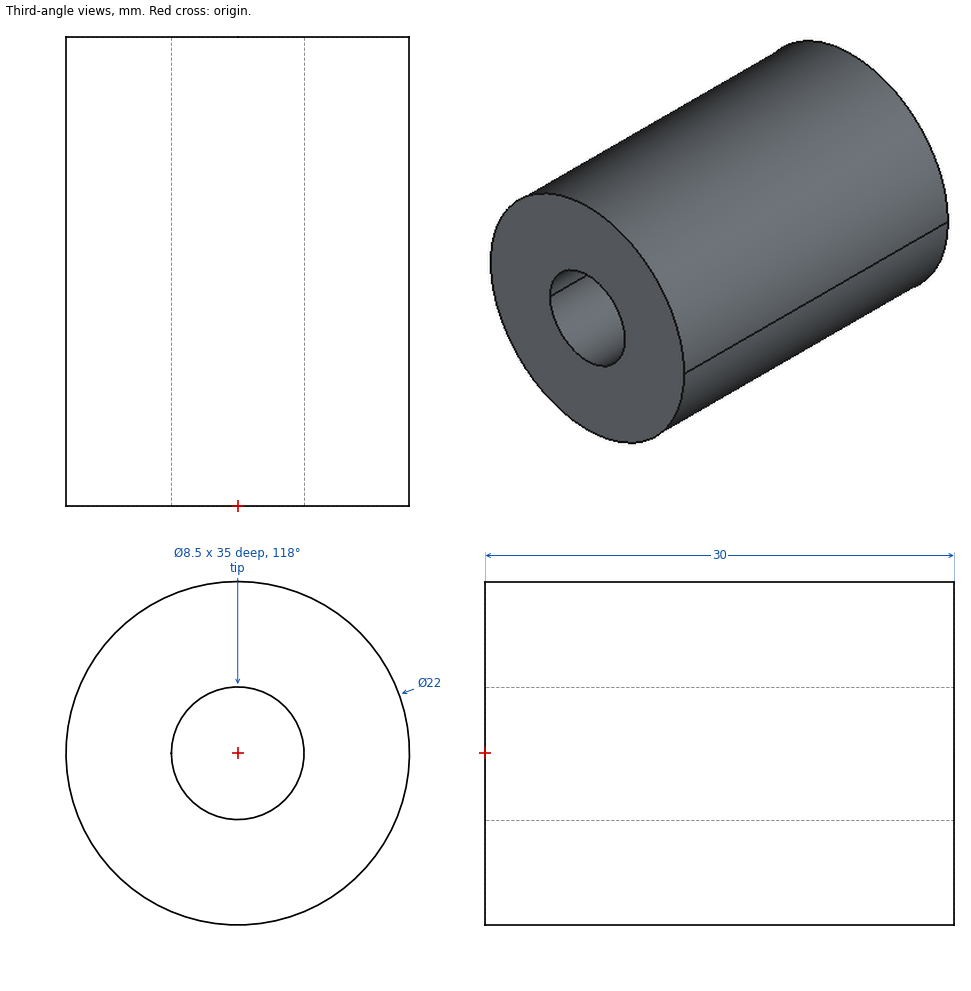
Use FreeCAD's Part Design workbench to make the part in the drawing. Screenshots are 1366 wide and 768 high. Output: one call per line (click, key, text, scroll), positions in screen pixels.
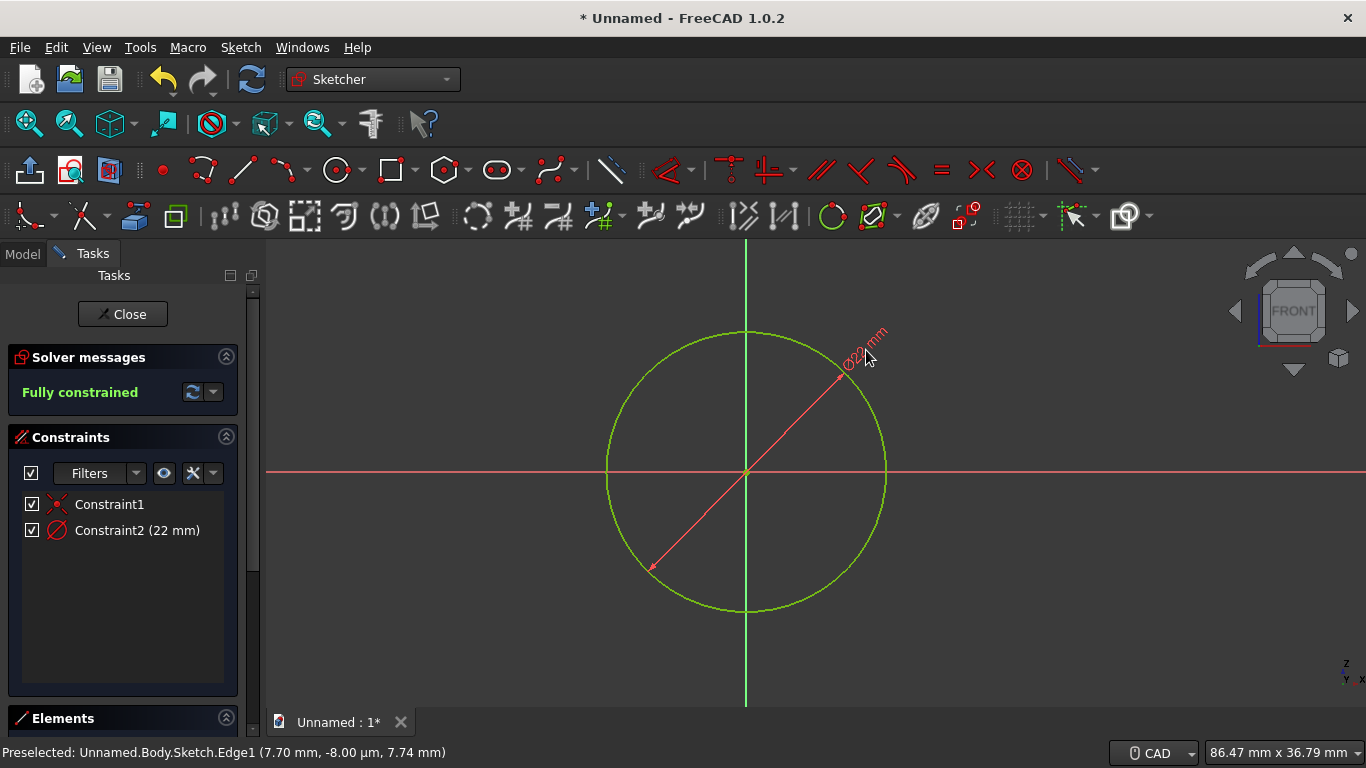
click(123, 314)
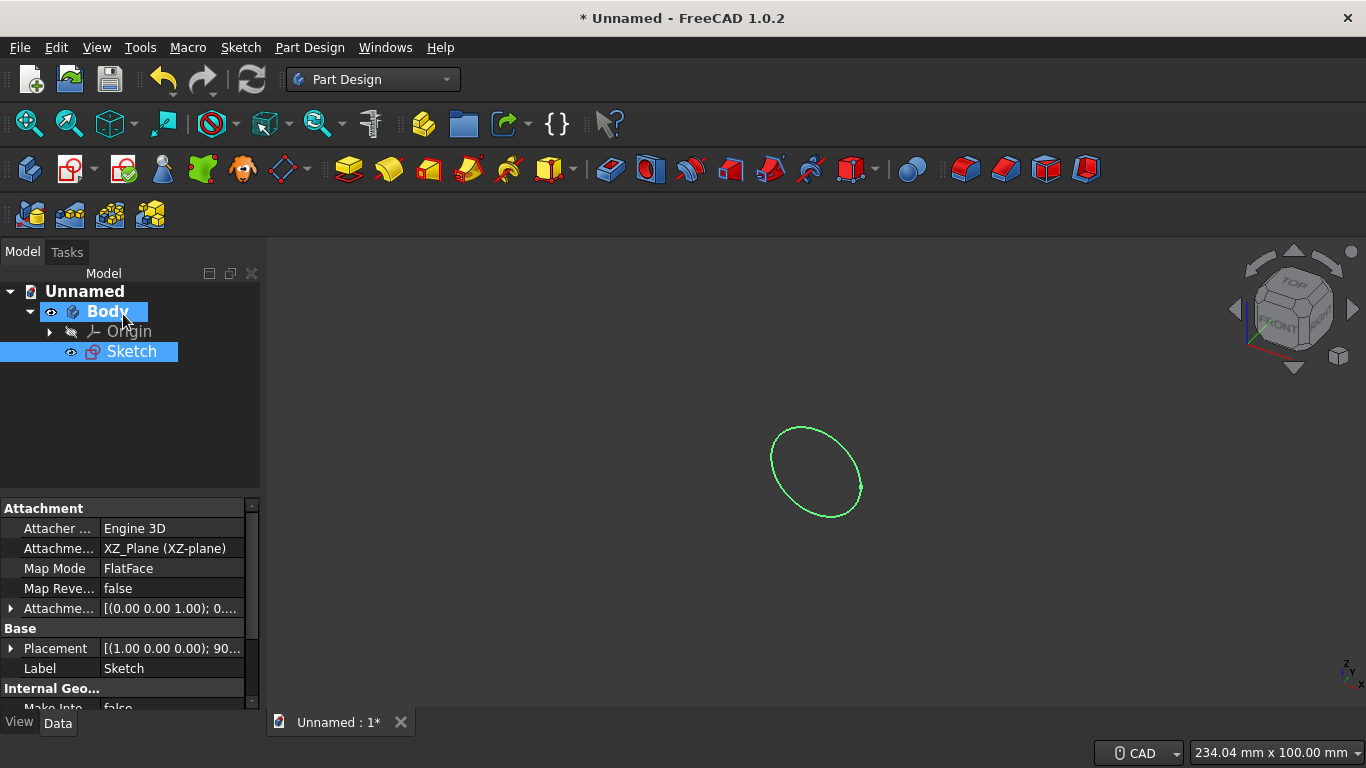
click(350, 170)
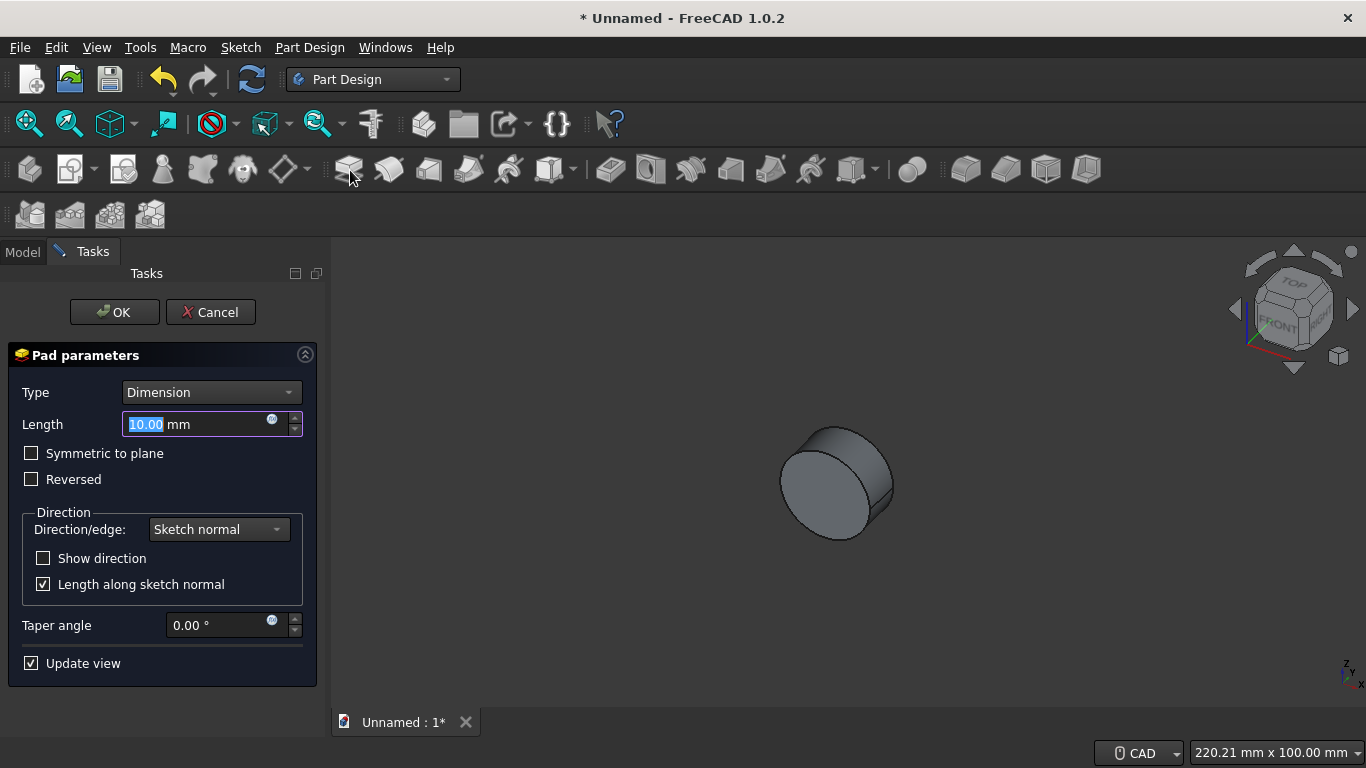
text(30)
key(Tab)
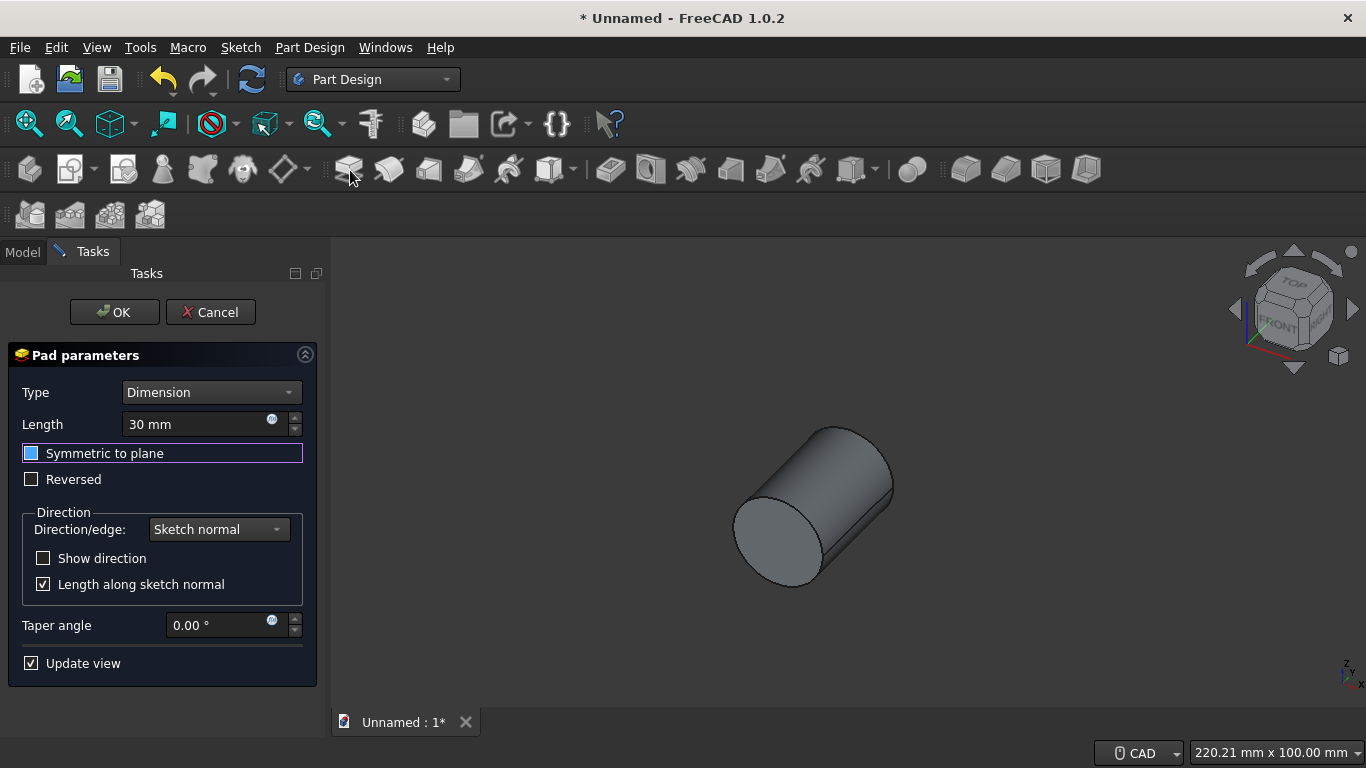
click(30, 479)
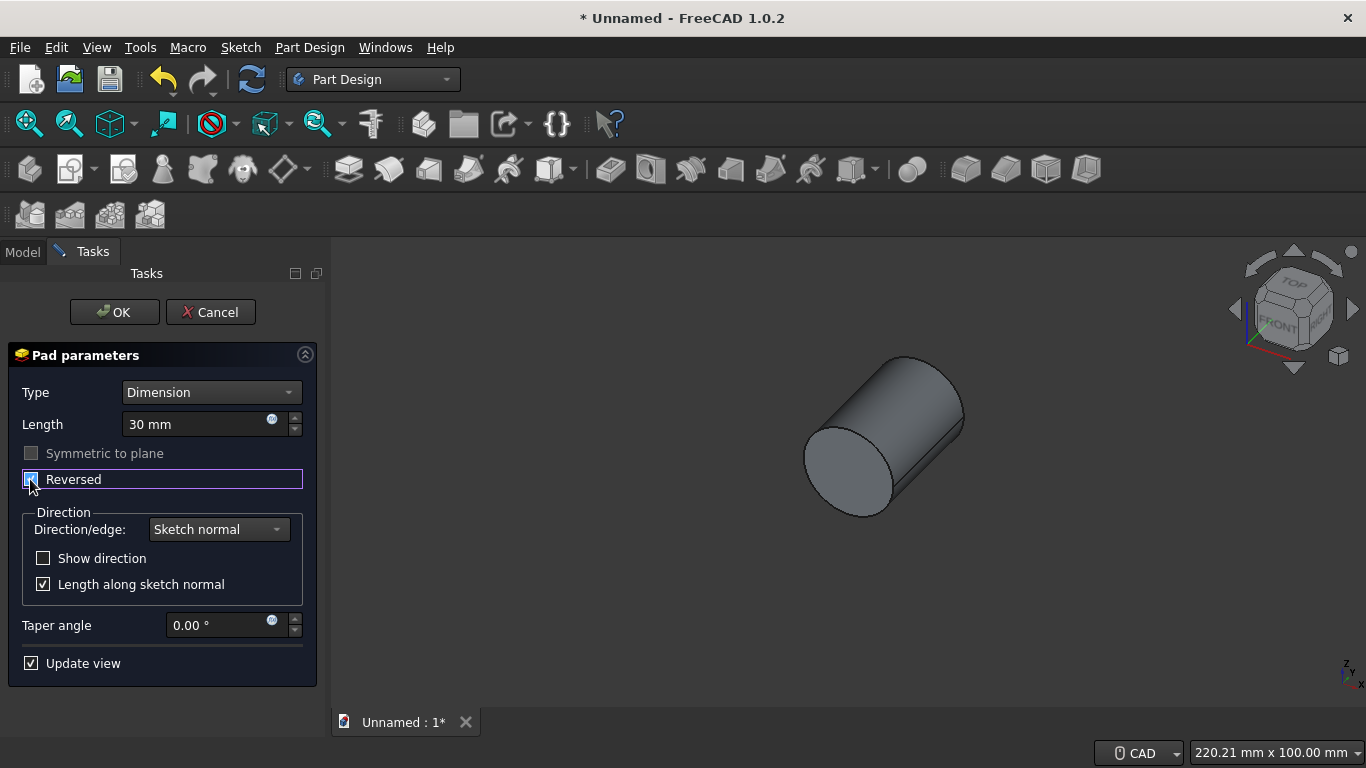
click(115, 312)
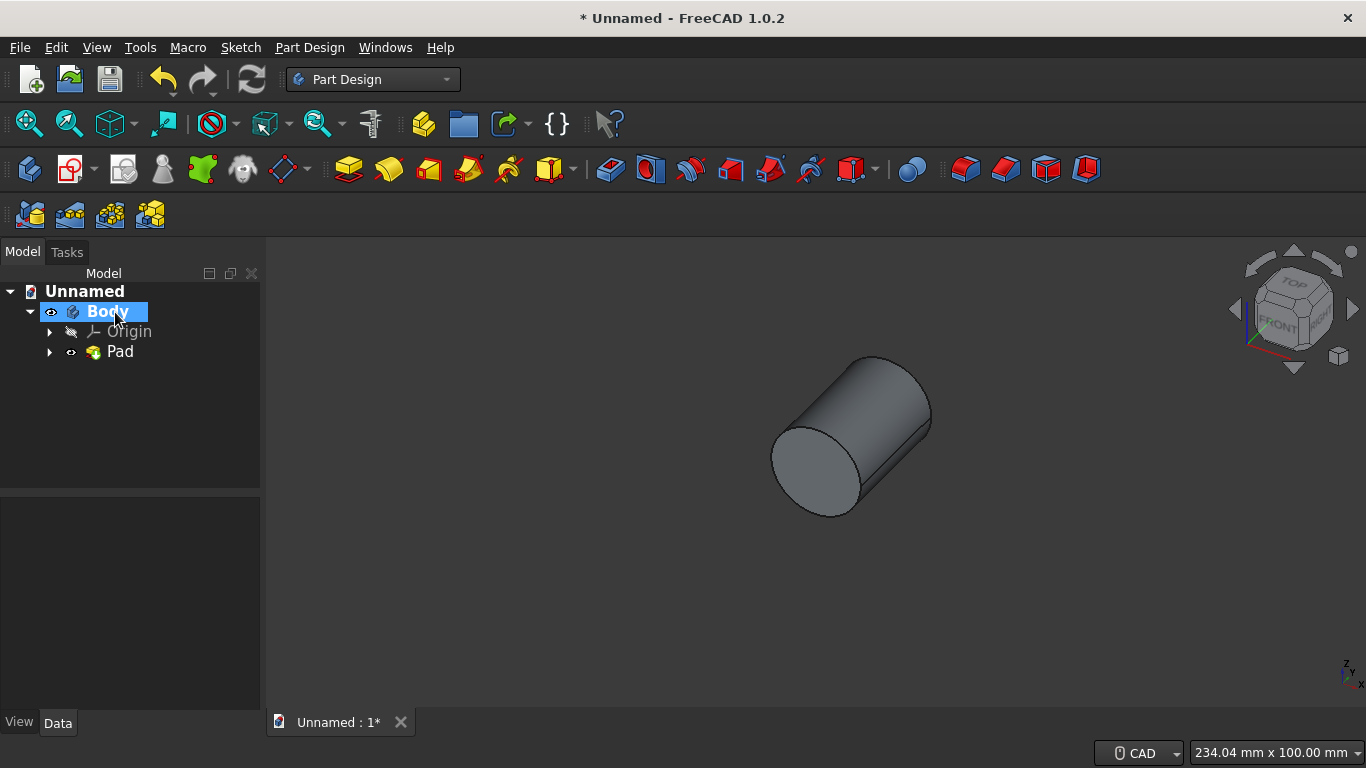
click(30, 124)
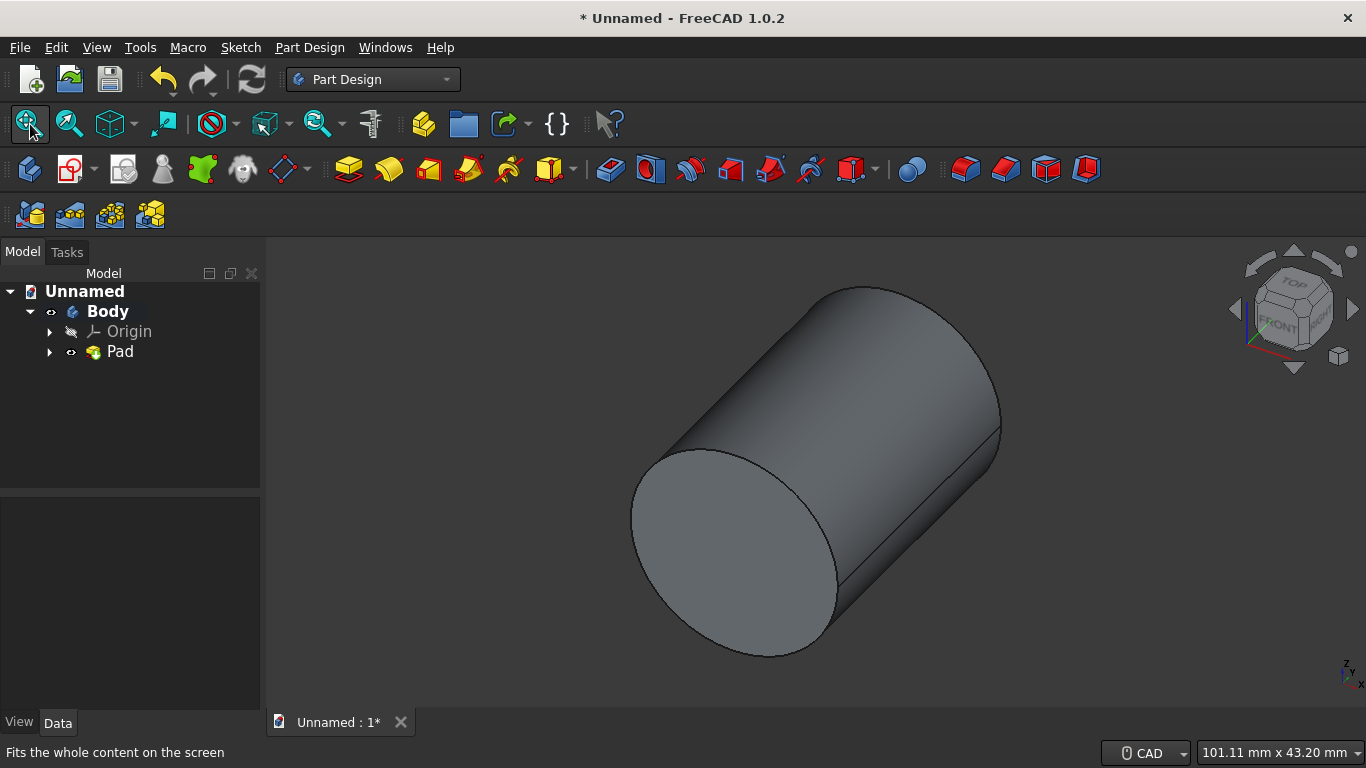
key(4)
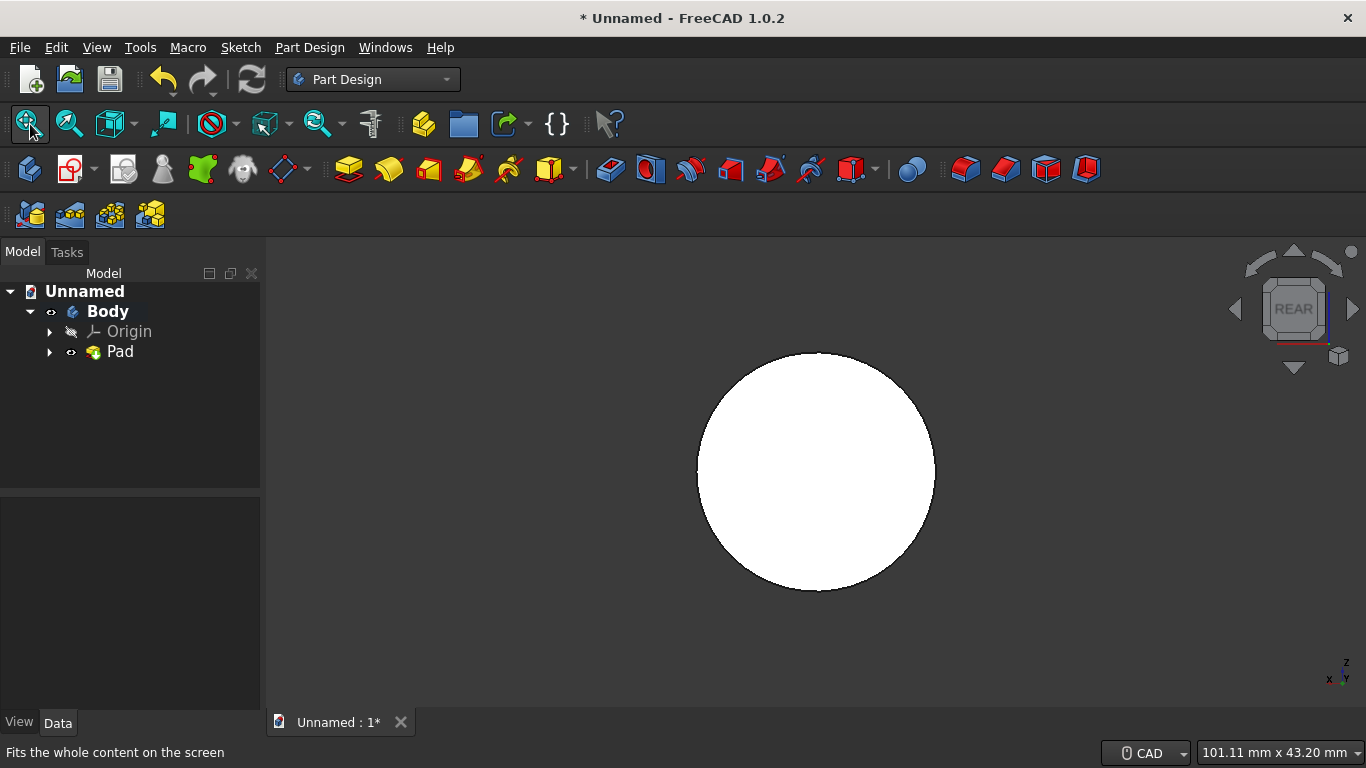
click(816, 471)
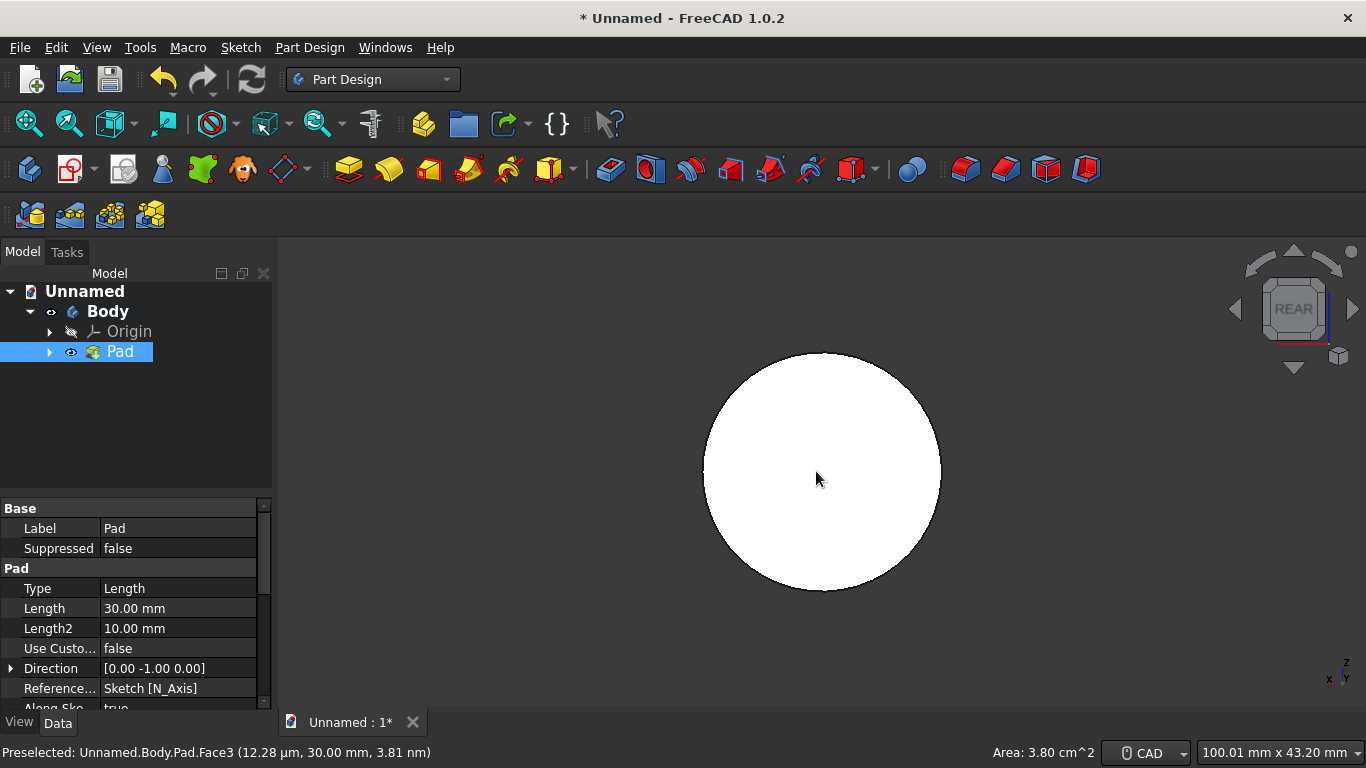
click(70, 170)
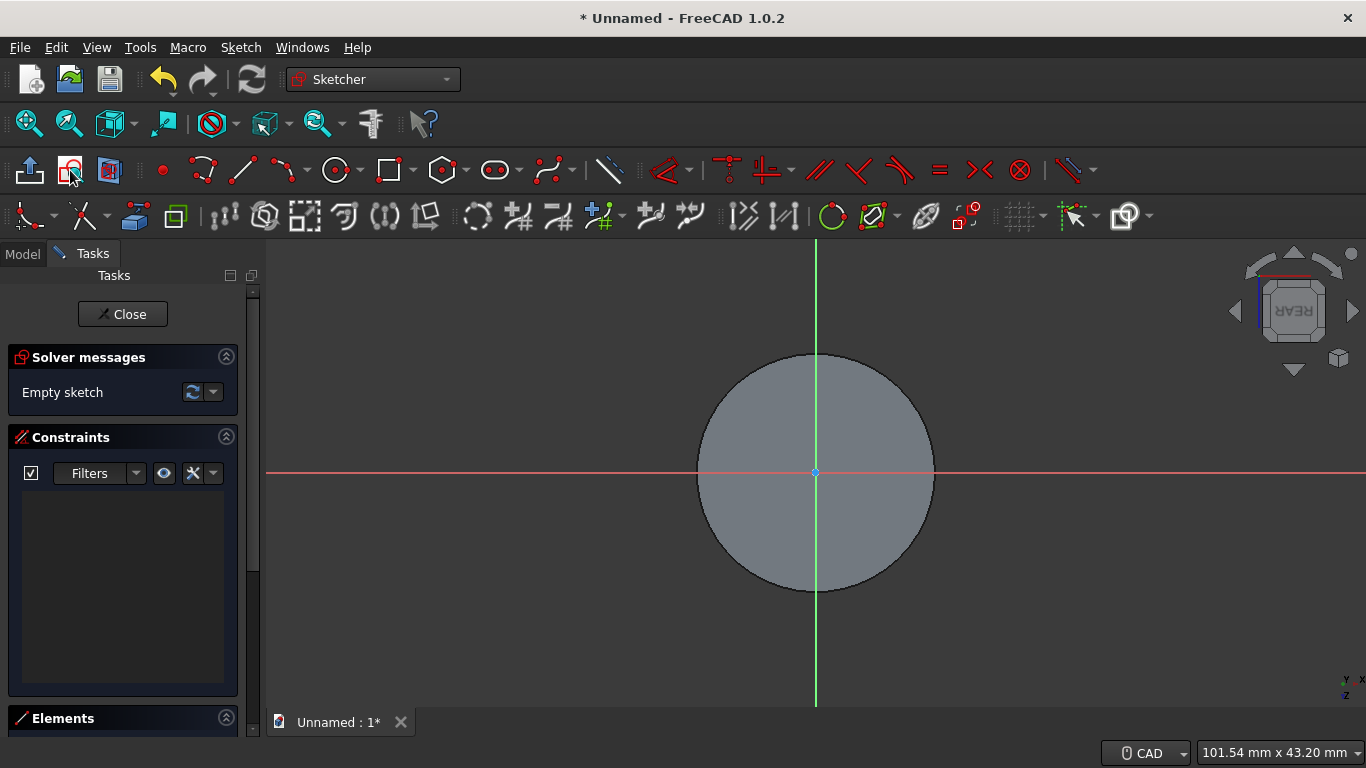
scroll(845, 473, up, 6)